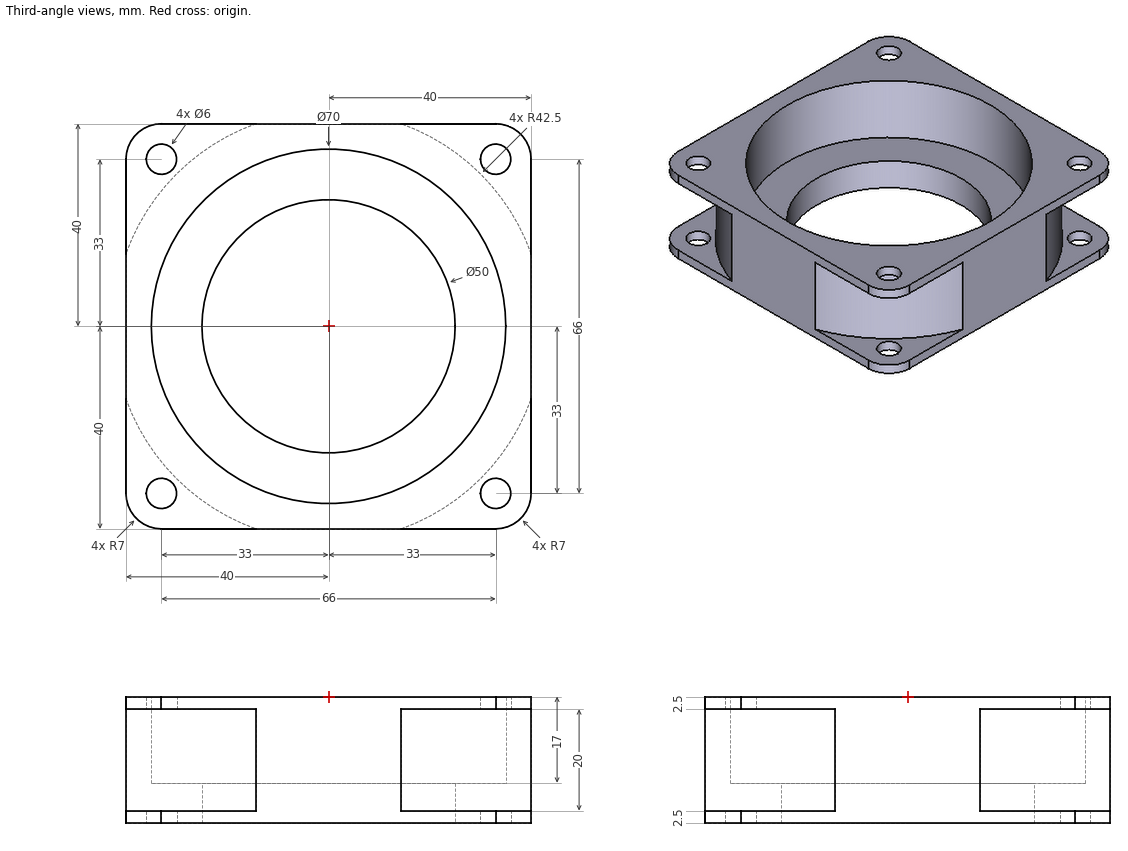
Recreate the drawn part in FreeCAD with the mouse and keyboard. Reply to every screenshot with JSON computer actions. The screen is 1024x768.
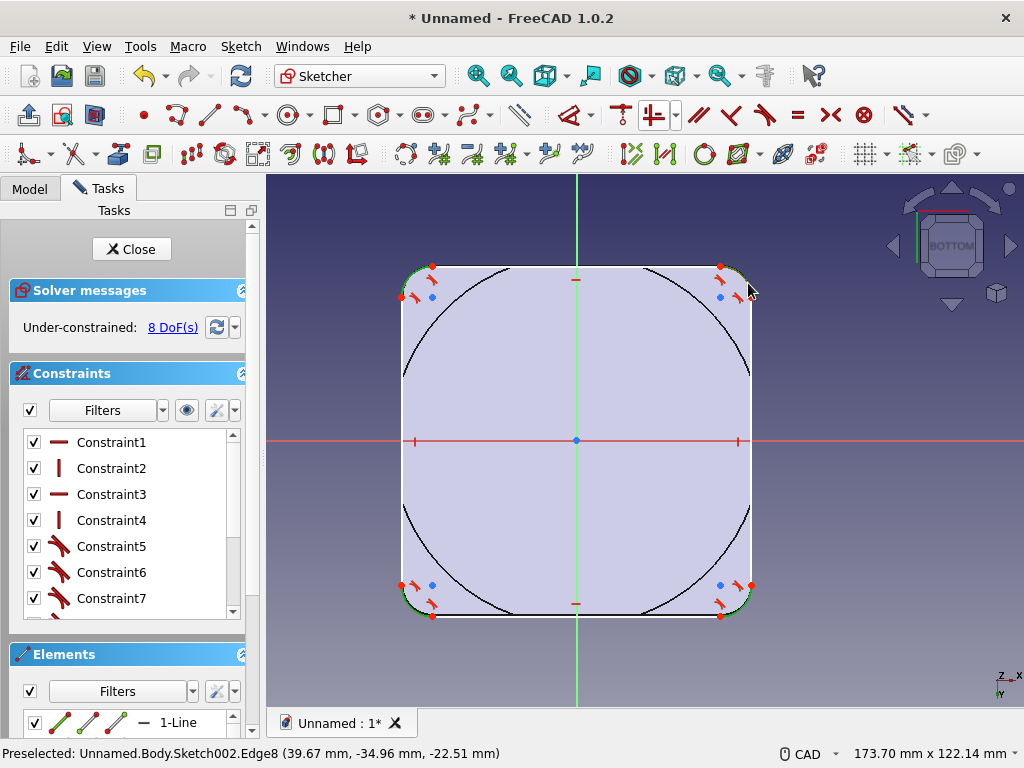
{"action": "left_click", "coordinate": [798, 116]}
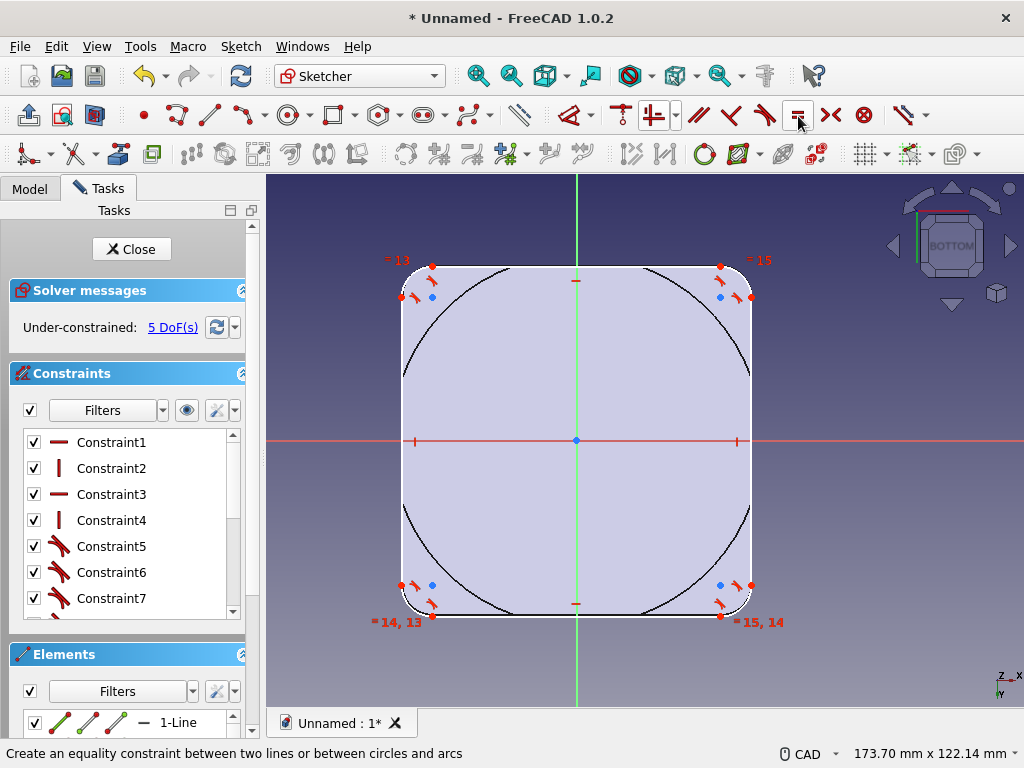
{"action": "left_click", "coordinate": [568, 116]}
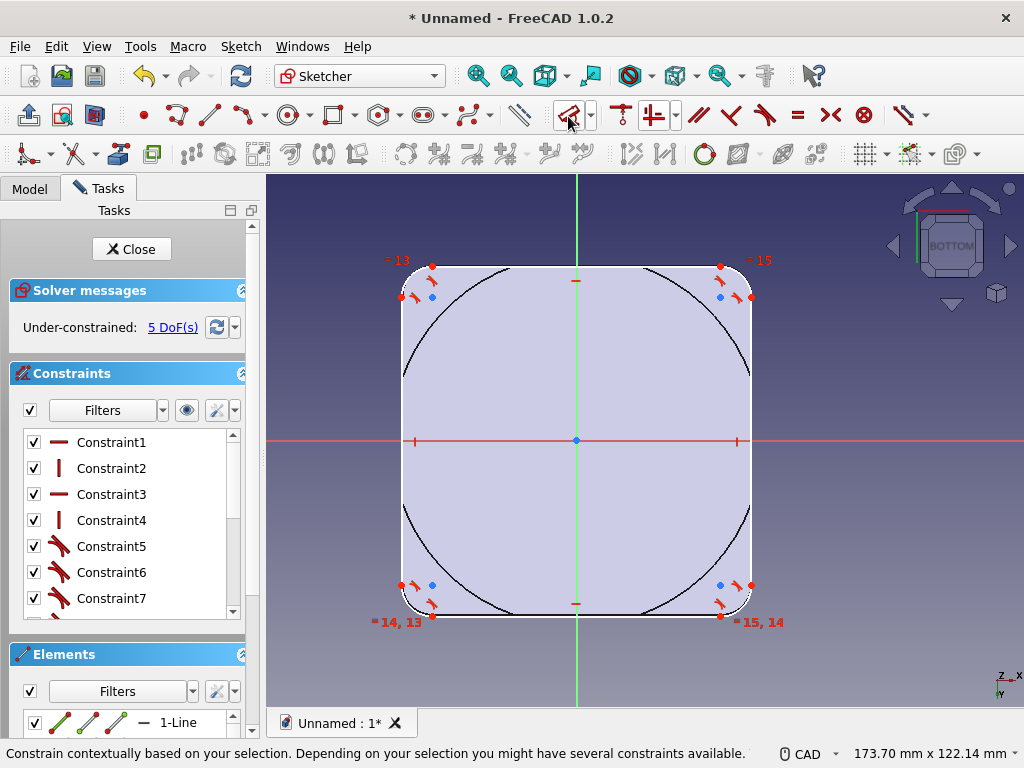
{"action": "scroll", "coordinate": [419, 270], "scroll_direction": "up", "scroll_amount": 2}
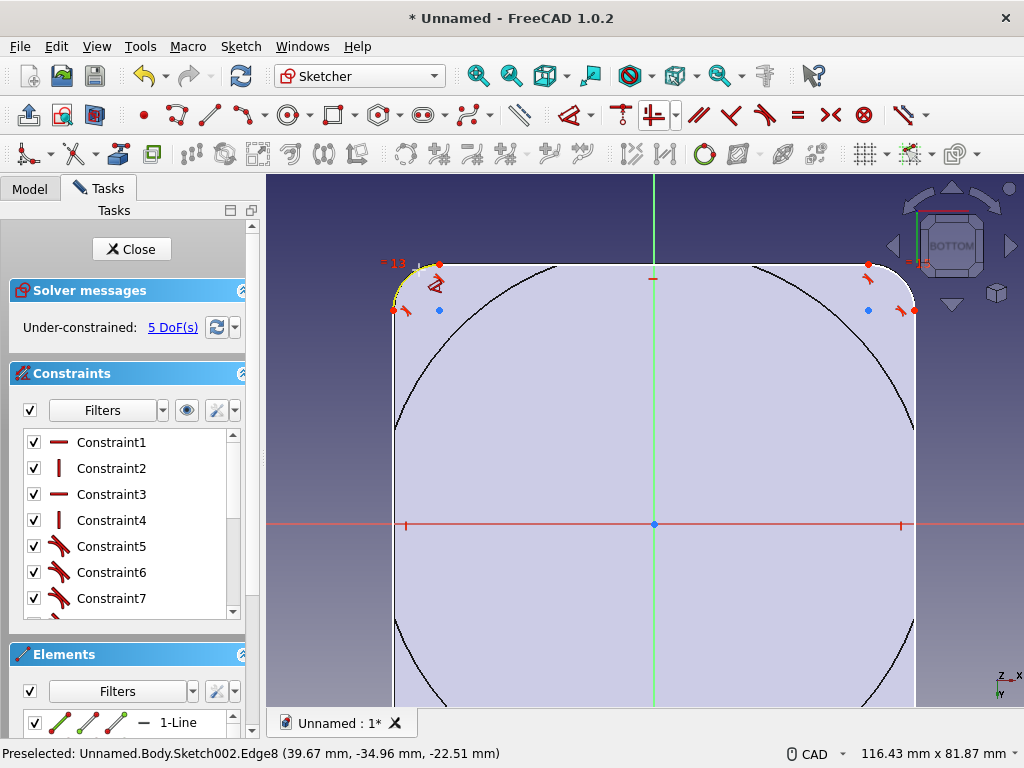
{"action": "left_click", "coordinate": [418, 270]}
{"action": "left_click", "coordinate": [403, 242]}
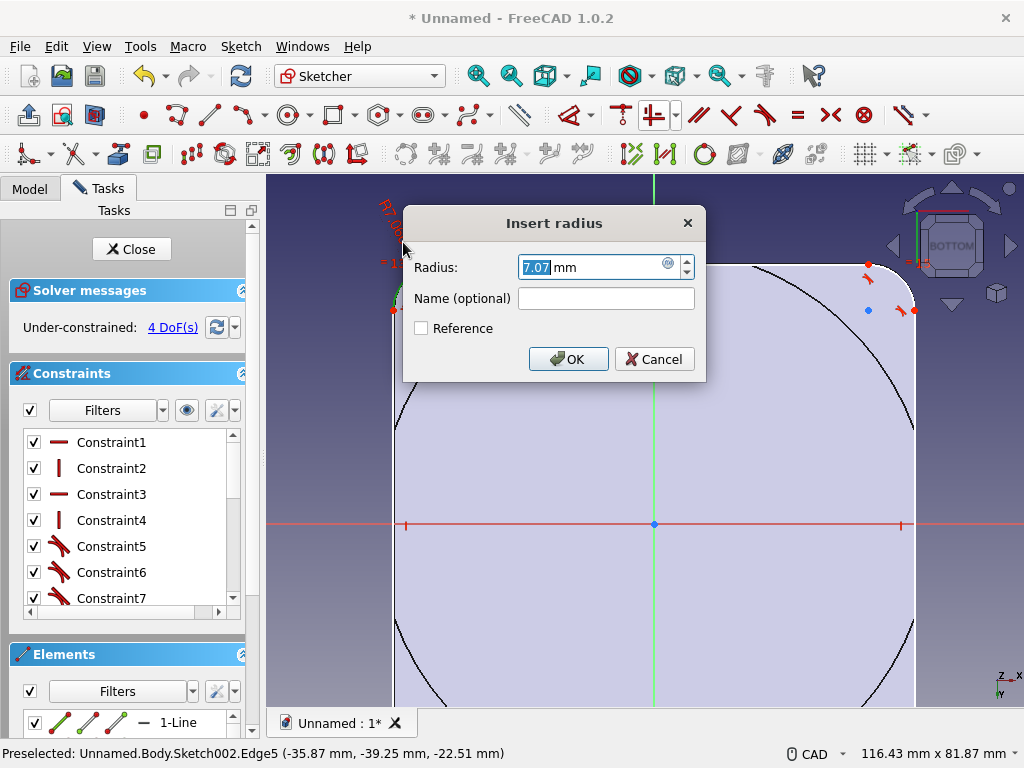
{"action": "type", "text": "7"}
{"action": "key", "text": "Return"}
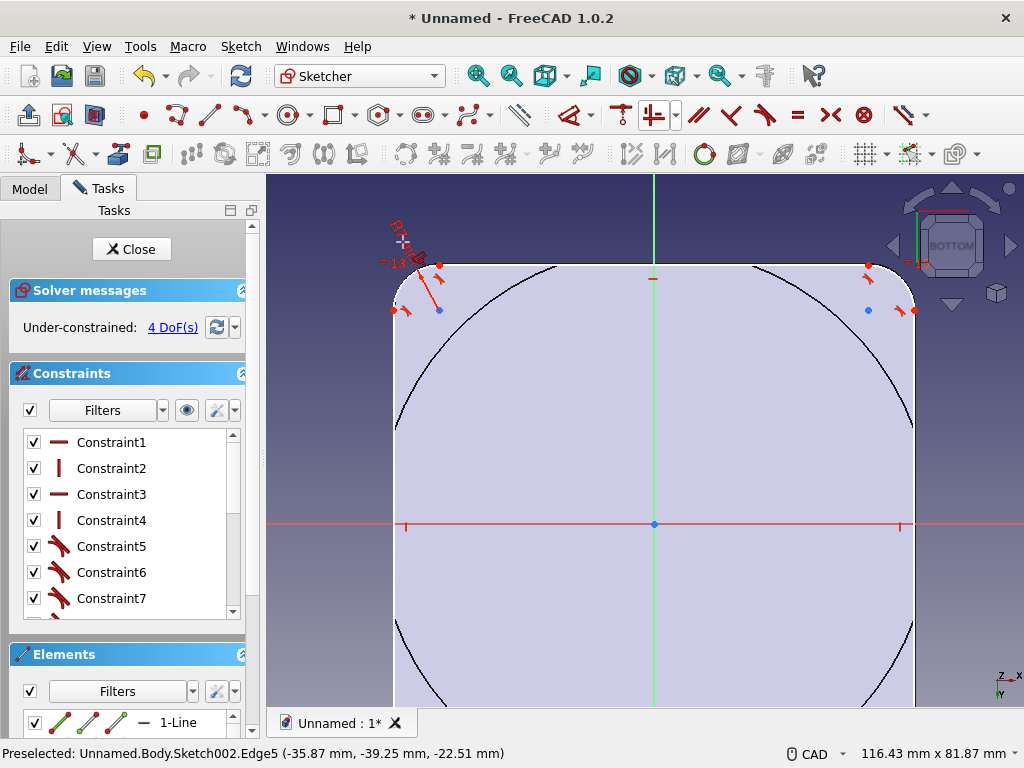
{"action": "left_click", "coordinate": [740, 265]}
{"action": "left_click", "coordinate": [553, 231]}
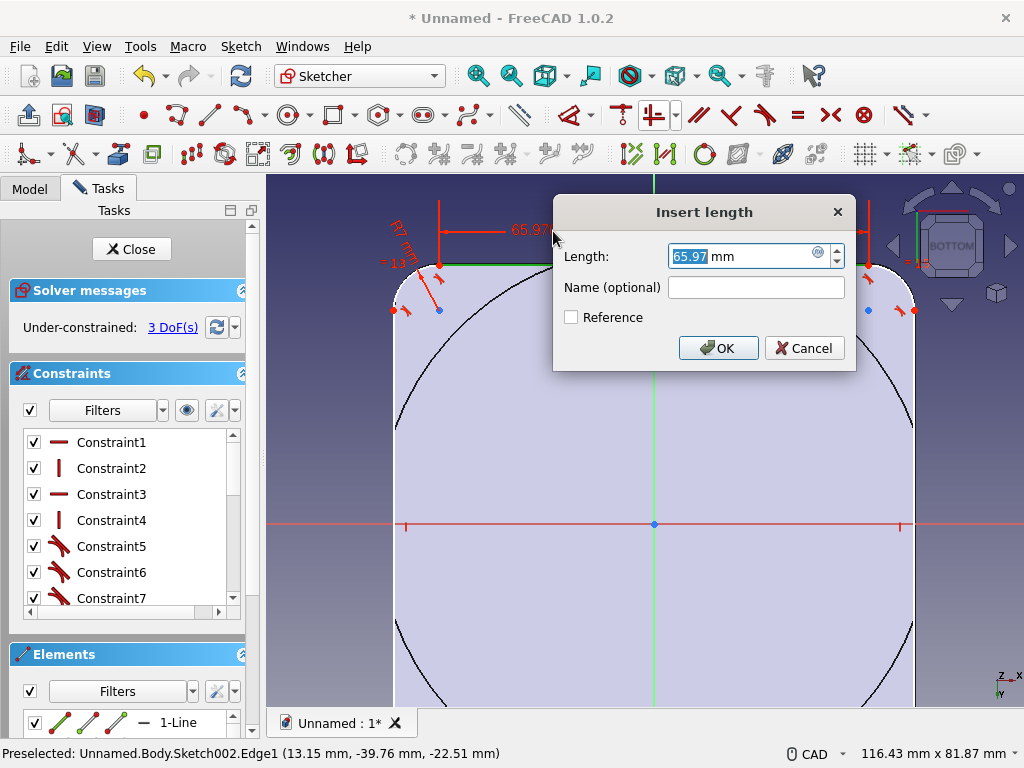
{"action": "type", "text": "66"}
{"action": "key", "text": "Return"}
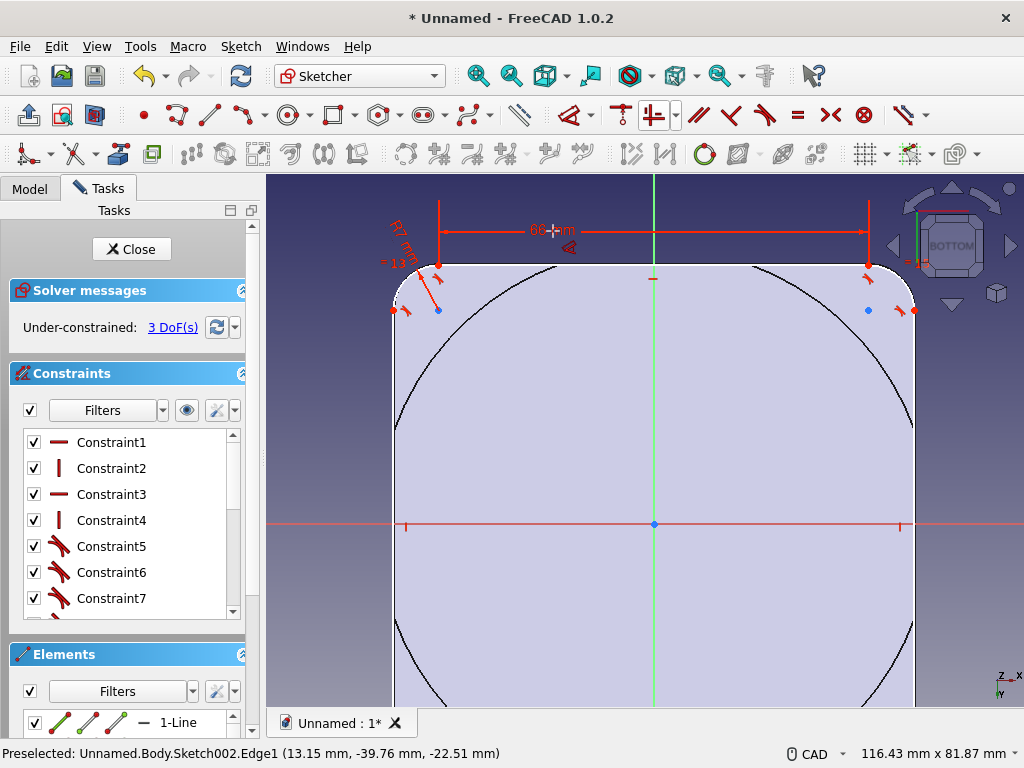
{"action": "left_click", "coordinate": [393, 440]}
{"action": "left_click", "coordinate": [359, 495]}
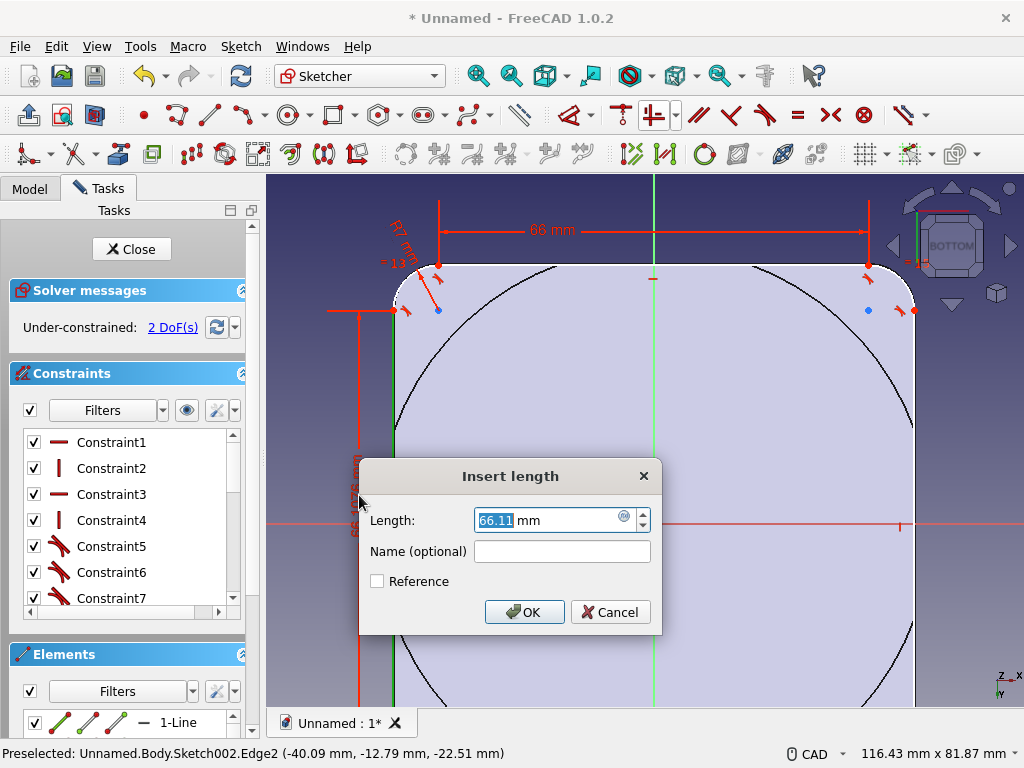
{"action": "type", "text": "66"}
{"action": "key", "text": "Return"}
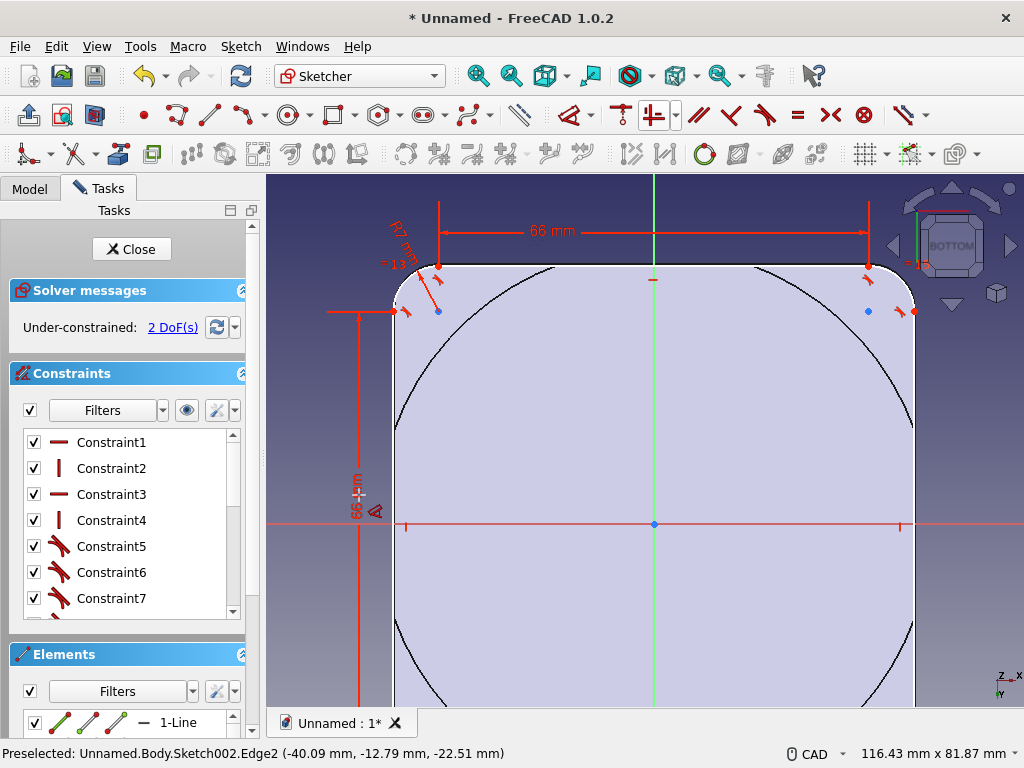
{"action": "scroll", "coordinate": [418, 270], "scroll_direction": "down", "scroll_amount": 2}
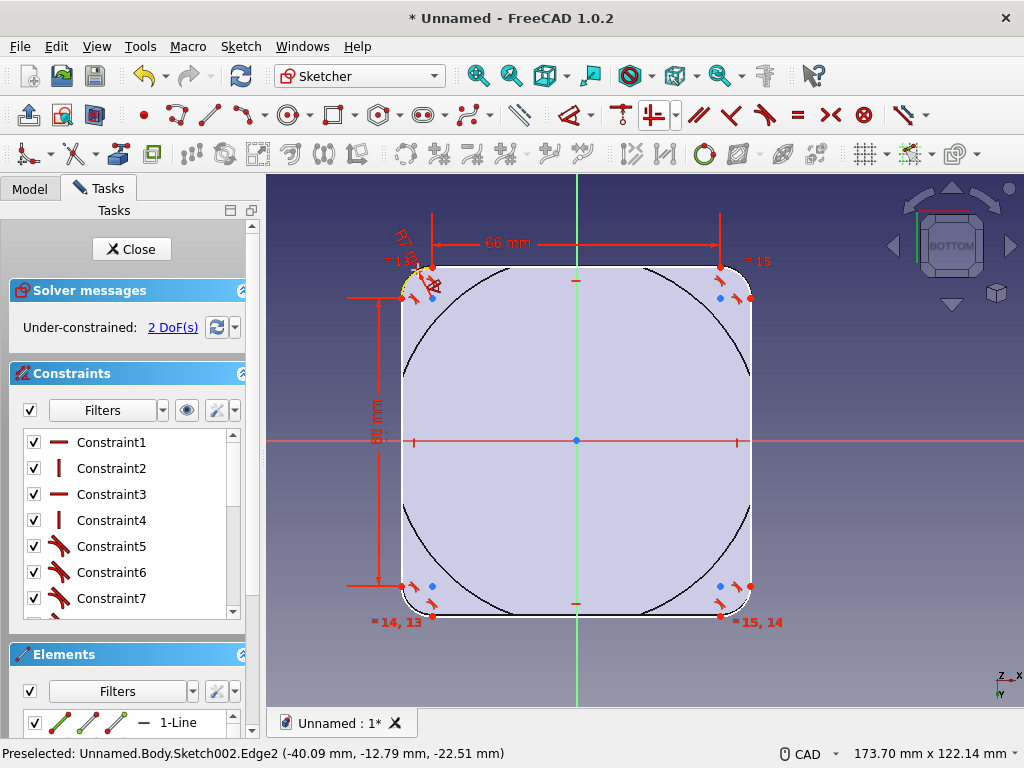
{"action": "left_click", "coordinate": [720, 267]}
{"action": "left_click", "coordinate": [648, 233]}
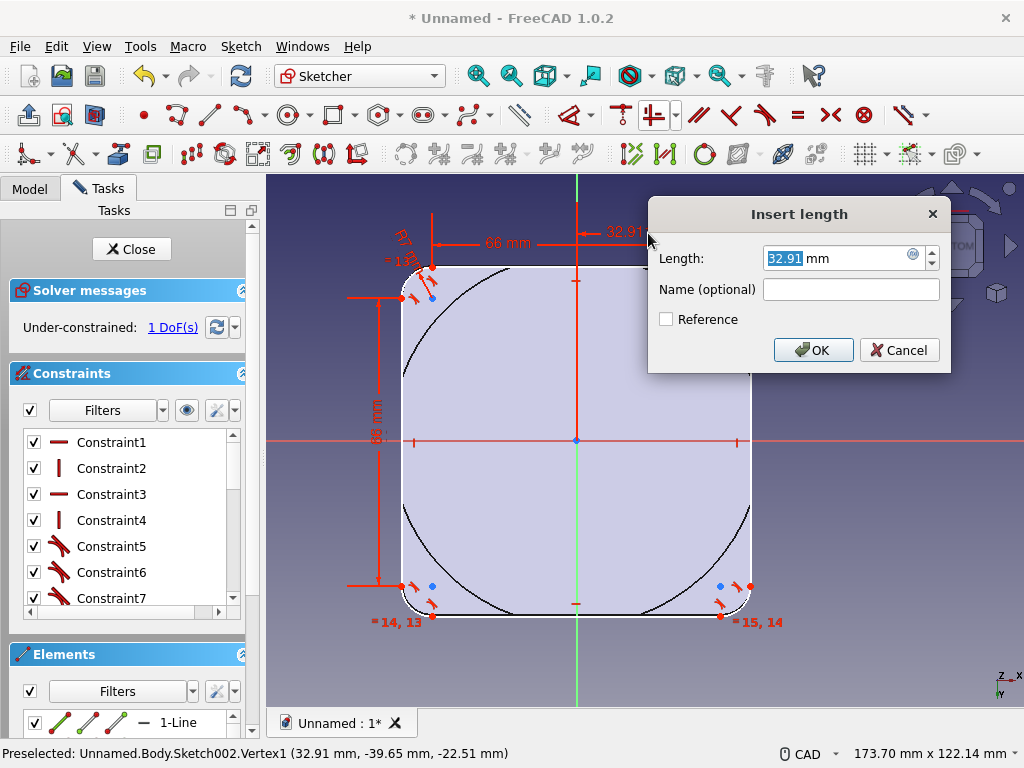
{"action": "type", "text": "33"}
{"action": "key", "text": "Return"}